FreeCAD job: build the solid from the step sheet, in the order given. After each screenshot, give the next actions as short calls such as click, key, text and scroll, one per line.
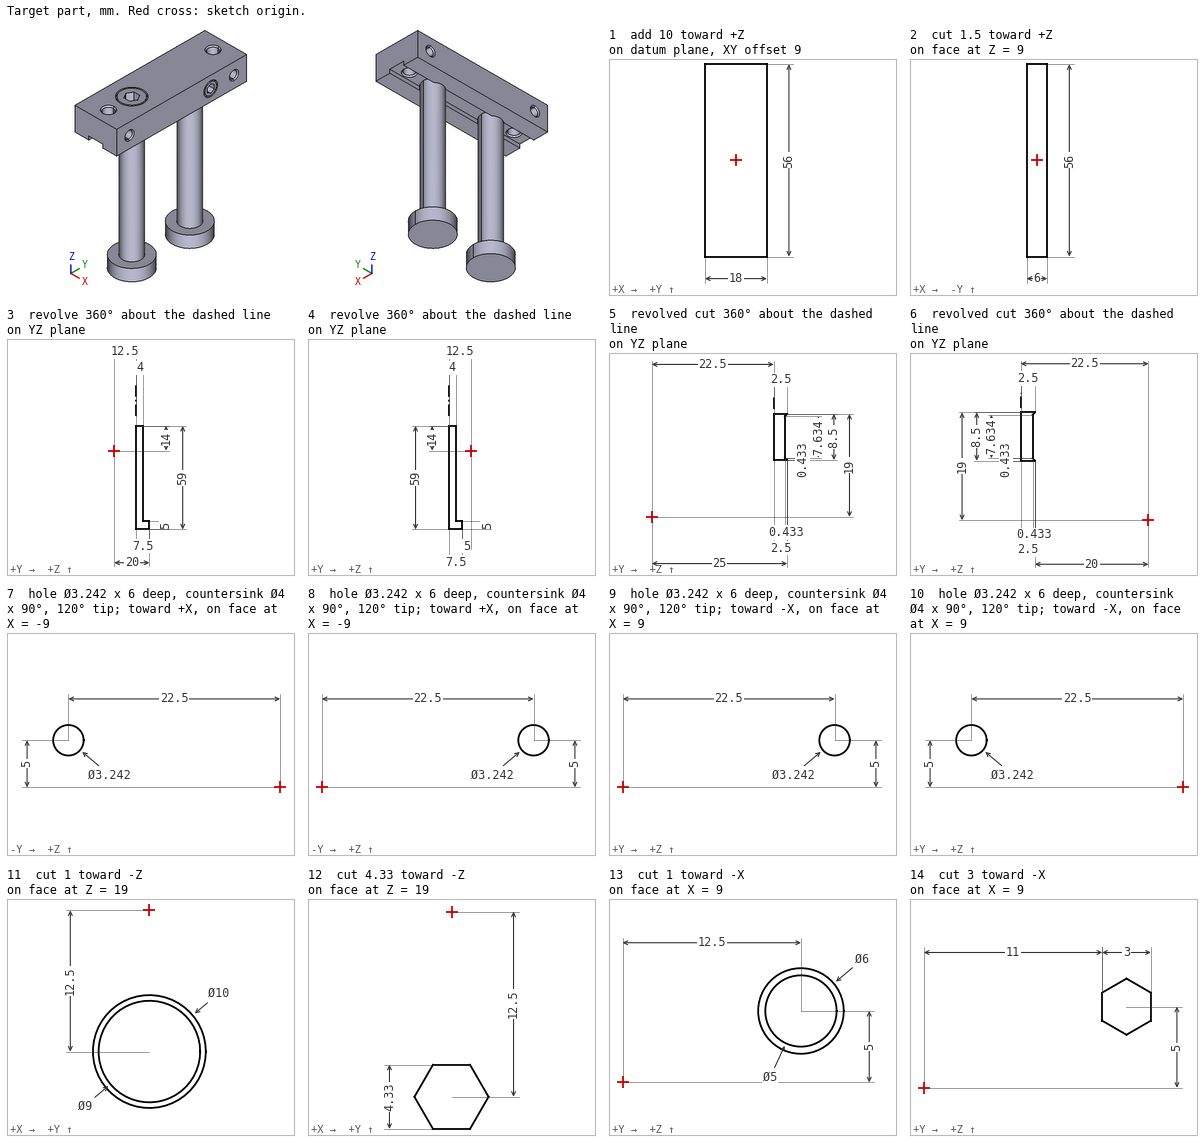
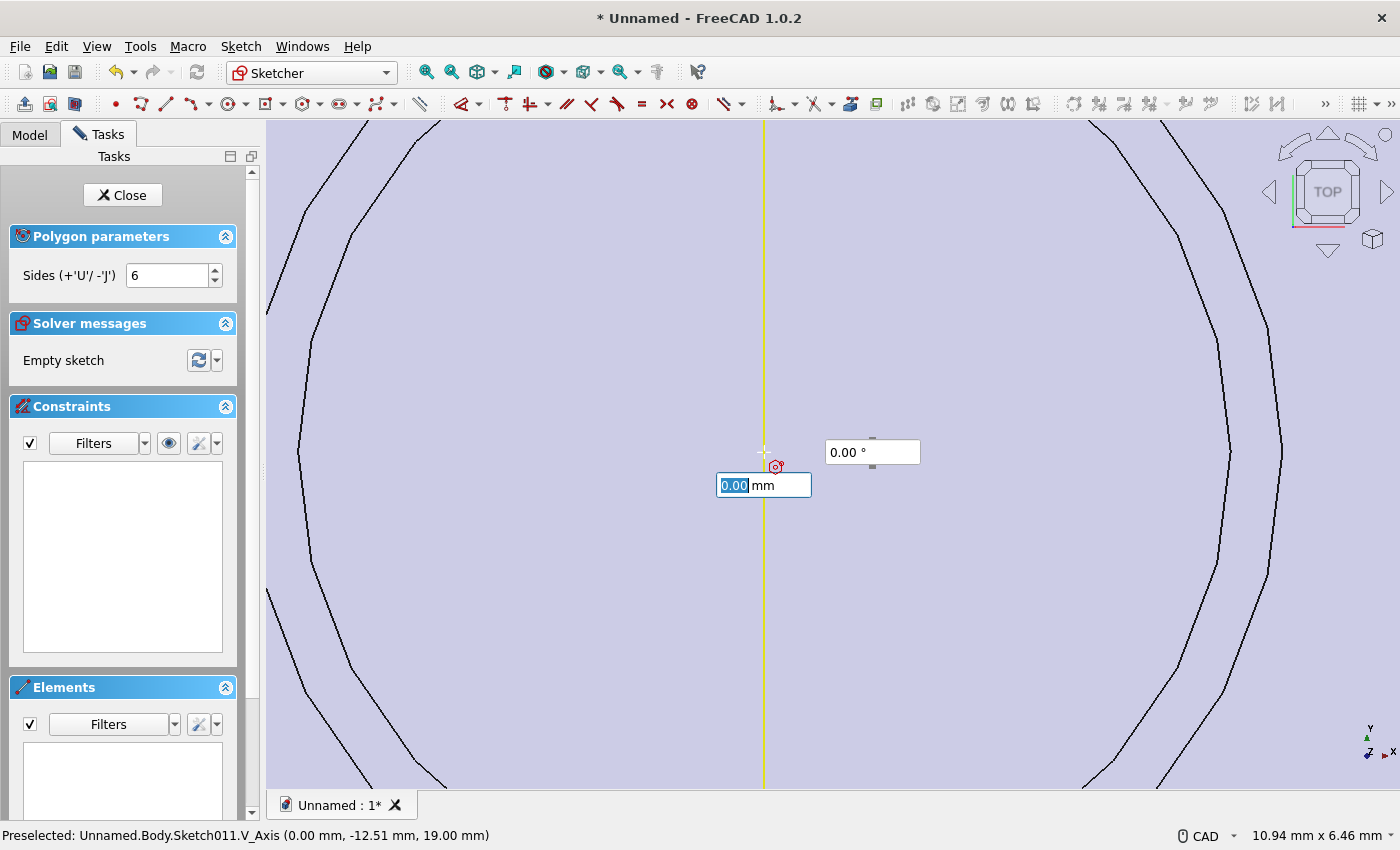
click(505, 452)
right_click(505, 452)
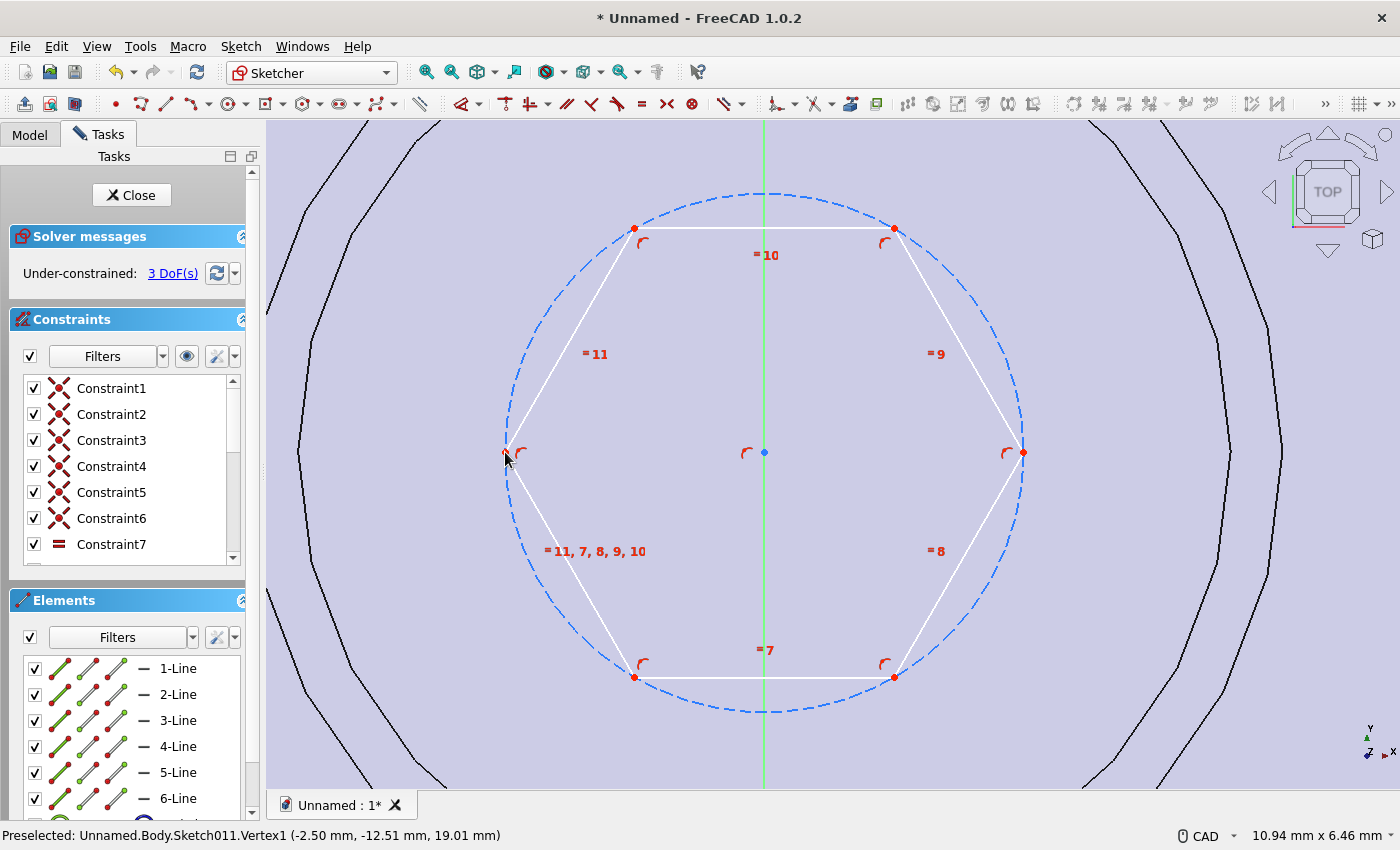
click(713, 678)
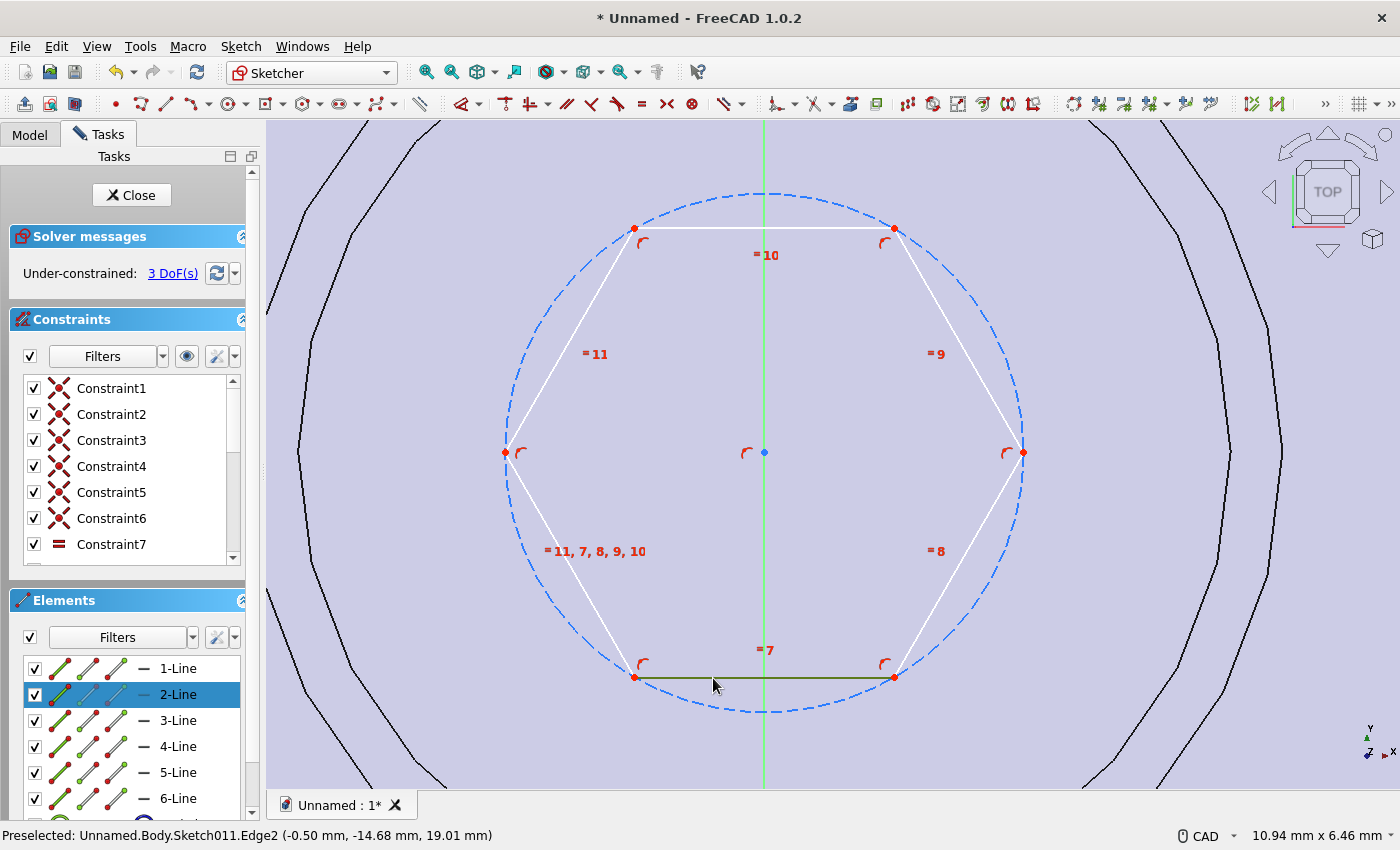
key(h)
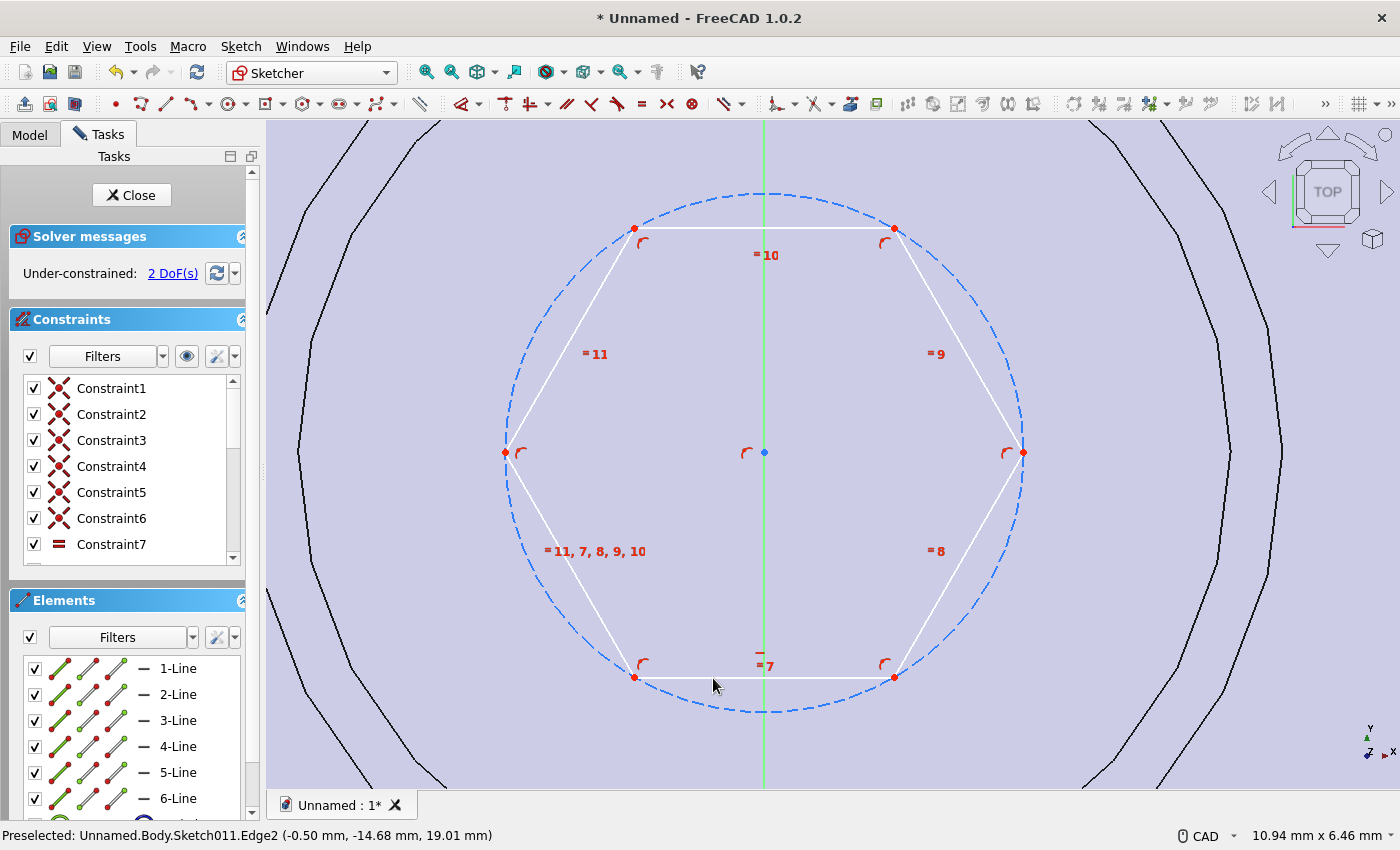
click(460, 104)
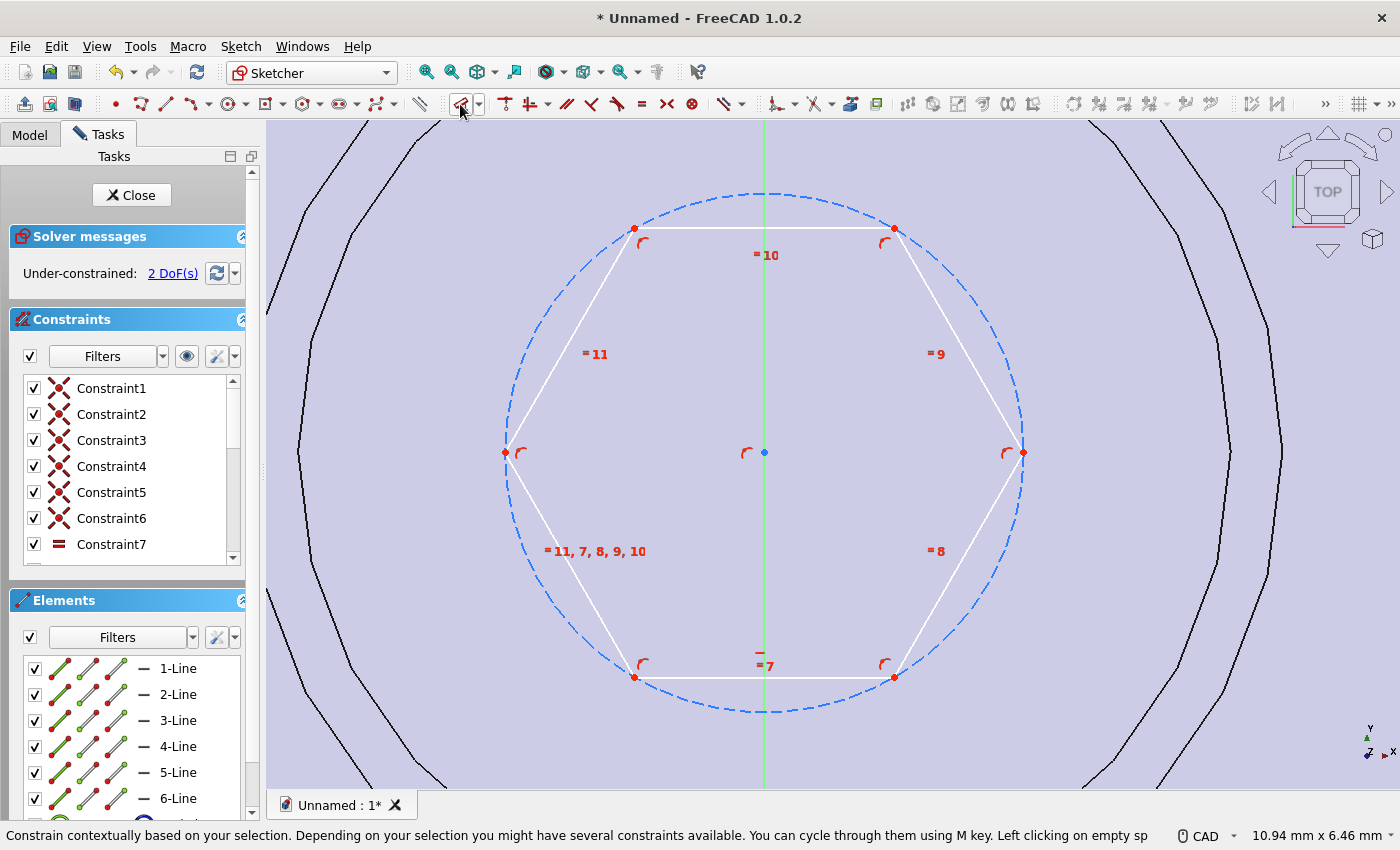
click(635, 678)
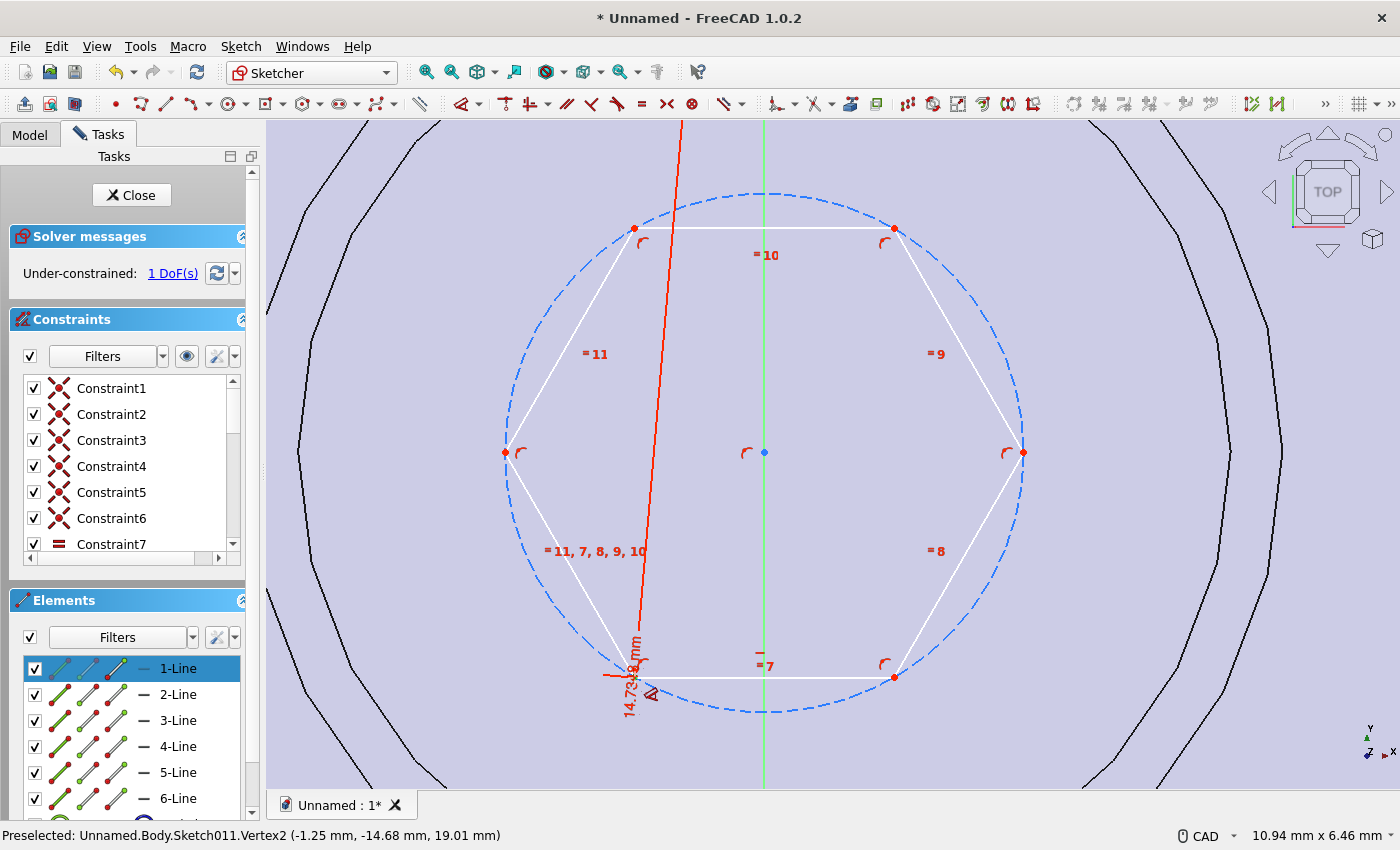
click(894, 228)
click(928, 453)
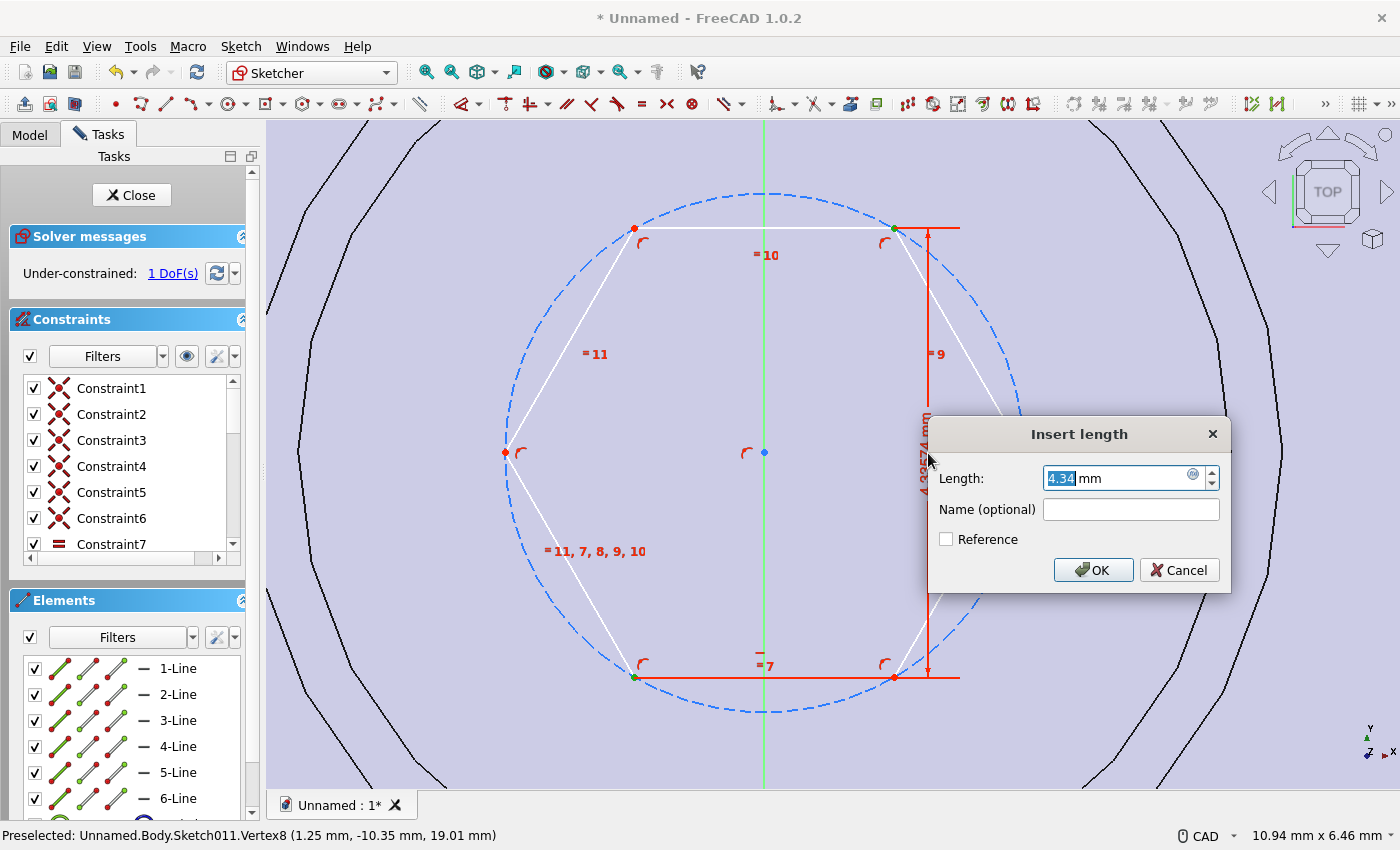
text(4.33)
key(Return)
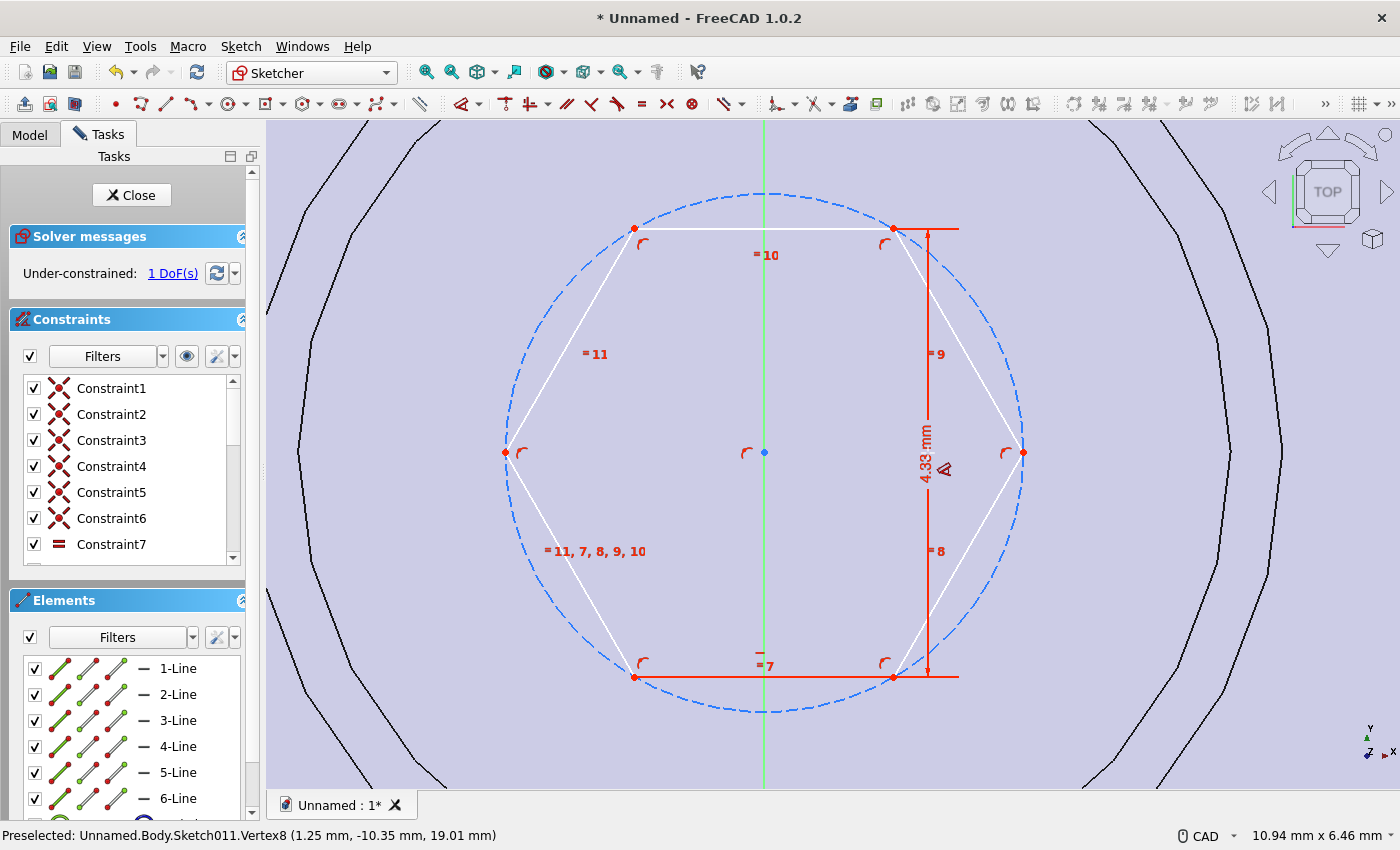
click(764, 453)
click(798, 301)